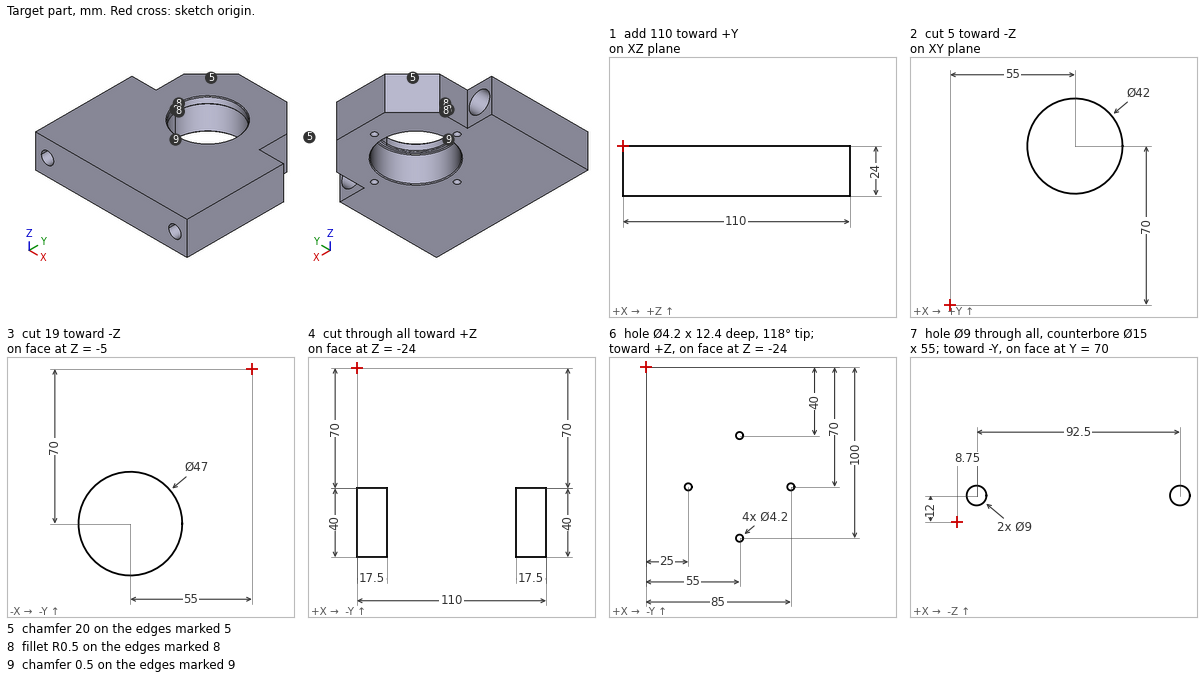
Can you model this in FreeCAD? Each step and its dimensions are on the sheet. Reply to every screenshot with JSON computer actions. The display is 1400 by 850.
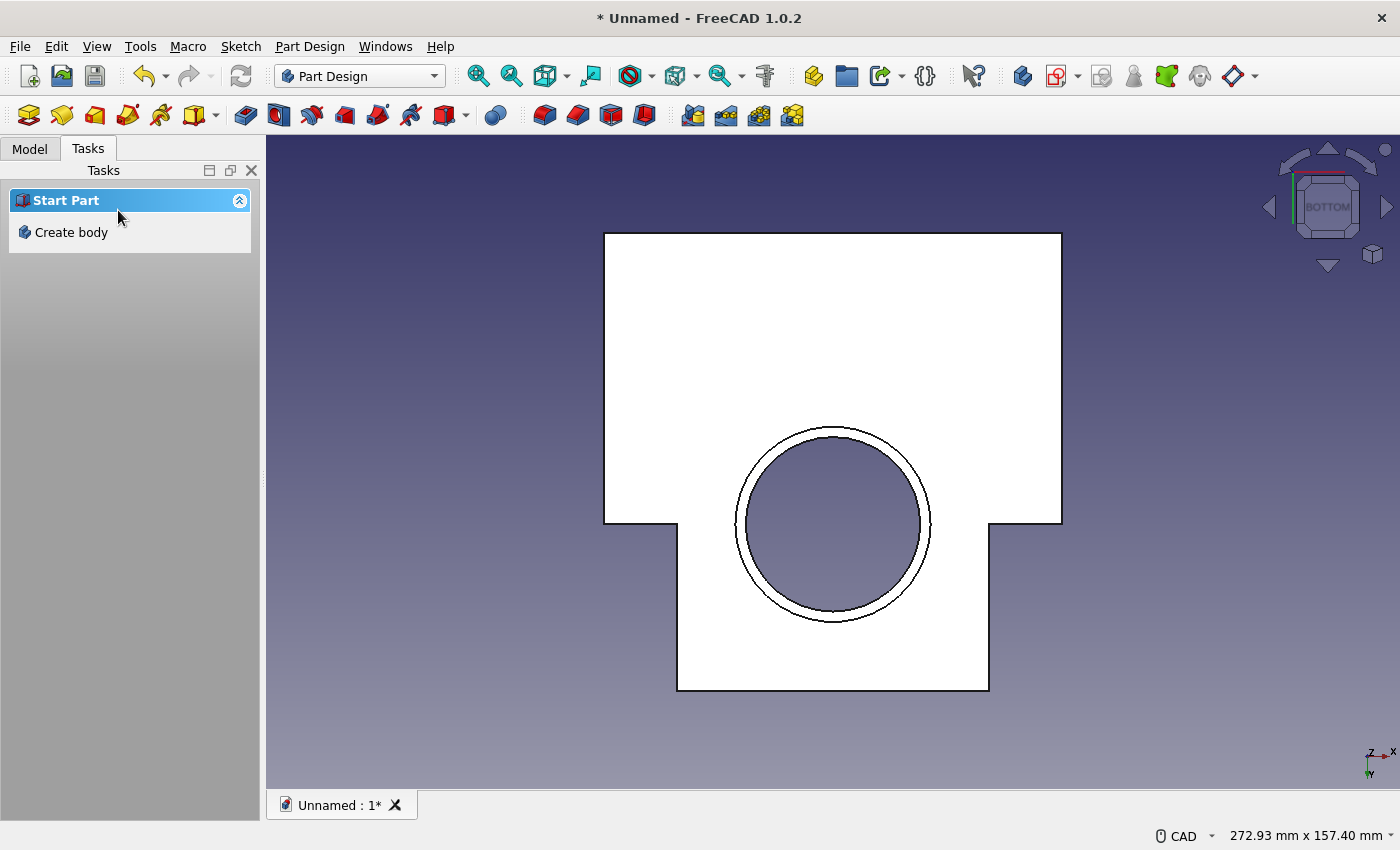
{"action": "key", "text": "0"}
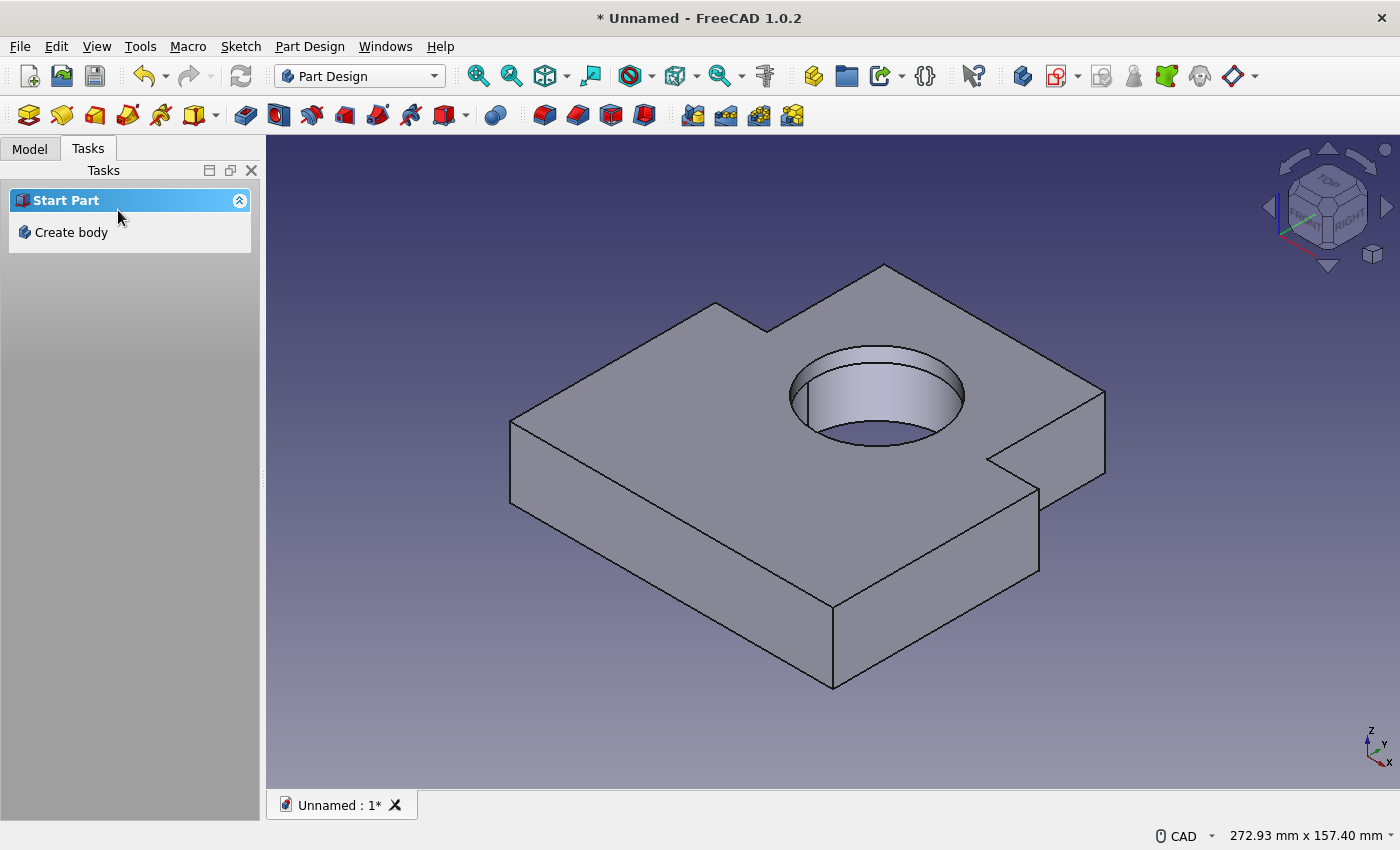
{"action": "key", "text": "2"}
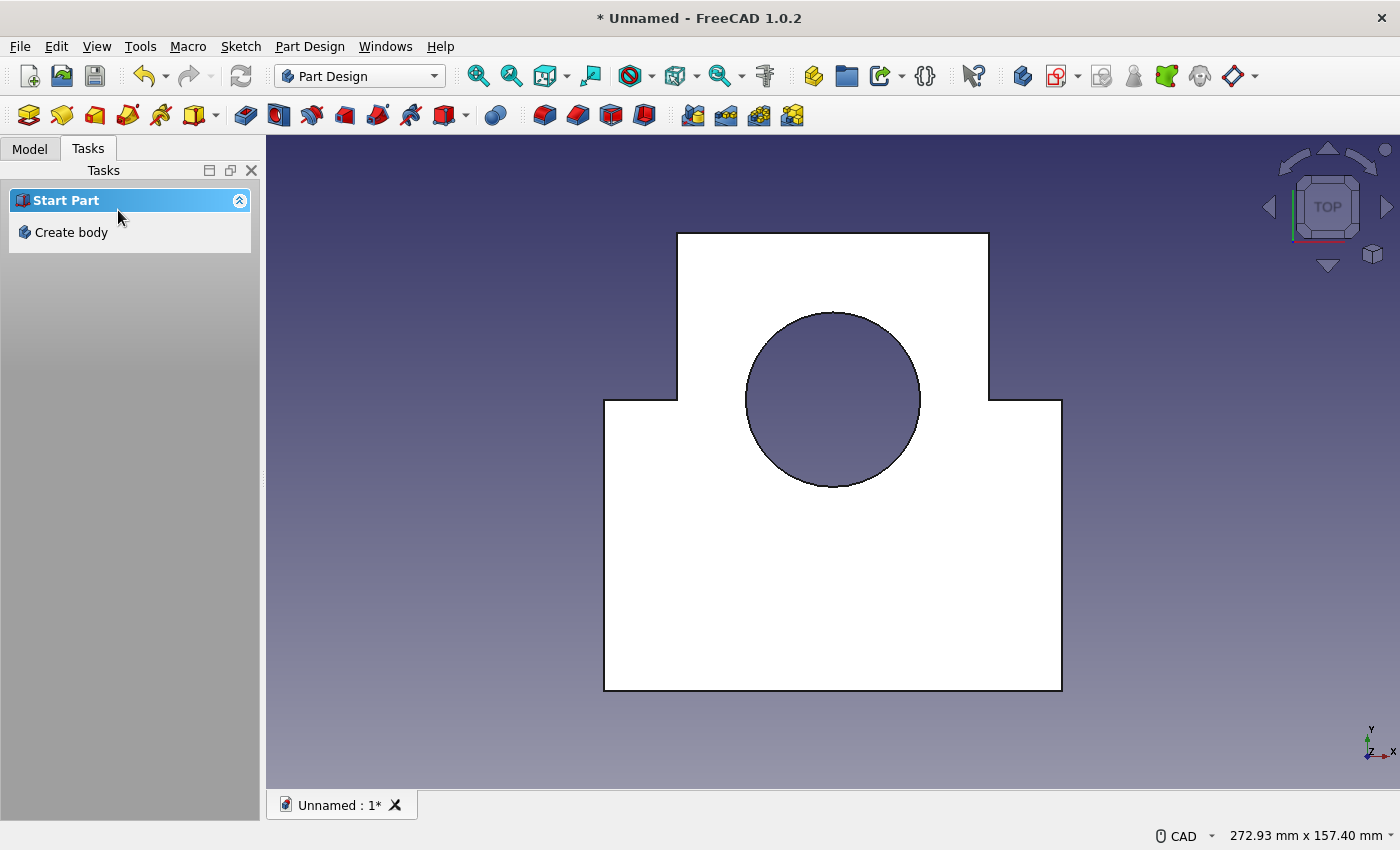
{"action": "key", "text": "1"}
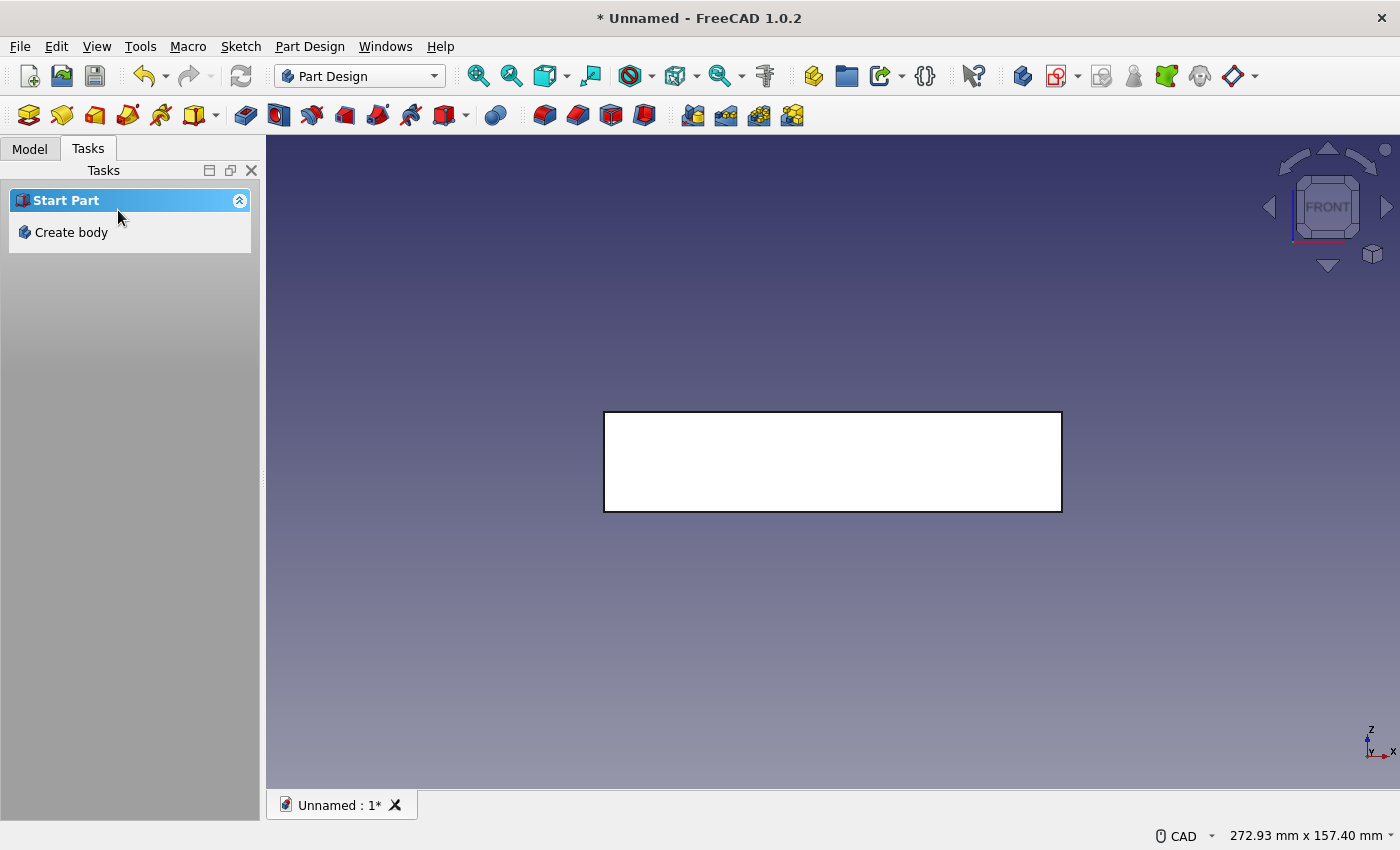
{"action": "left_click", "coordinate": [479, 76]}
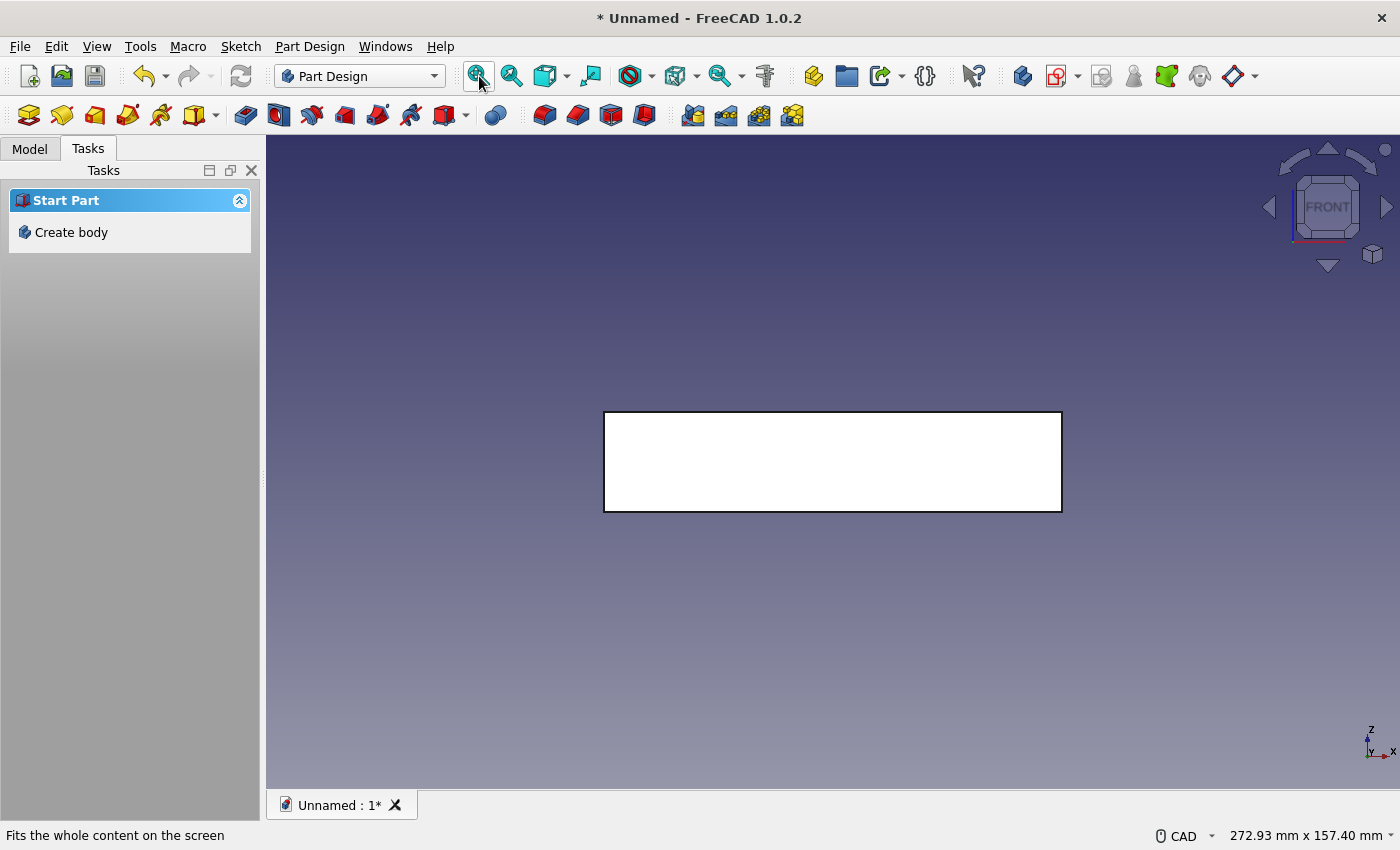
{"action": "key", "text": "3"}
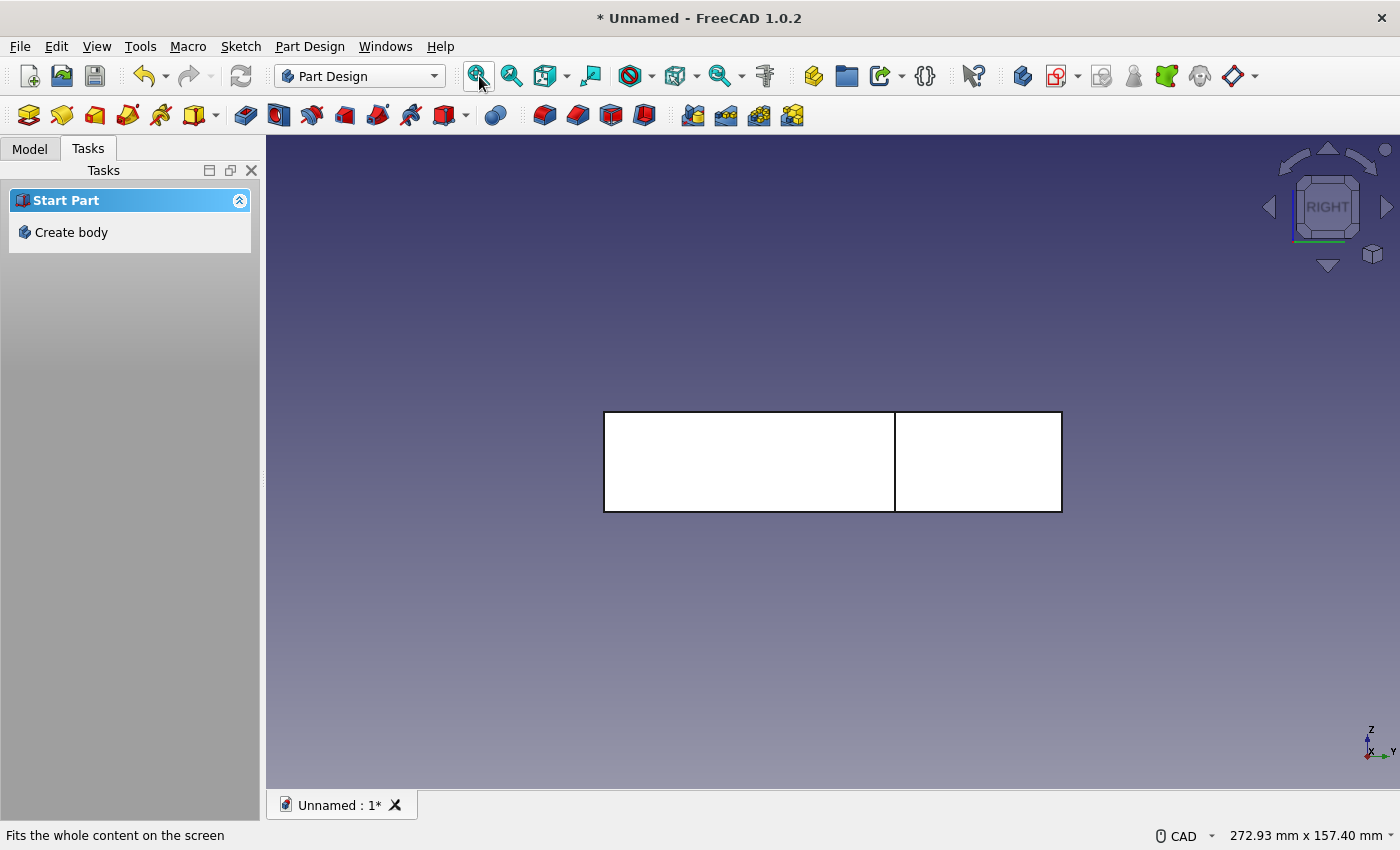
{"action": "left_click", "coordinate": [479, 76]}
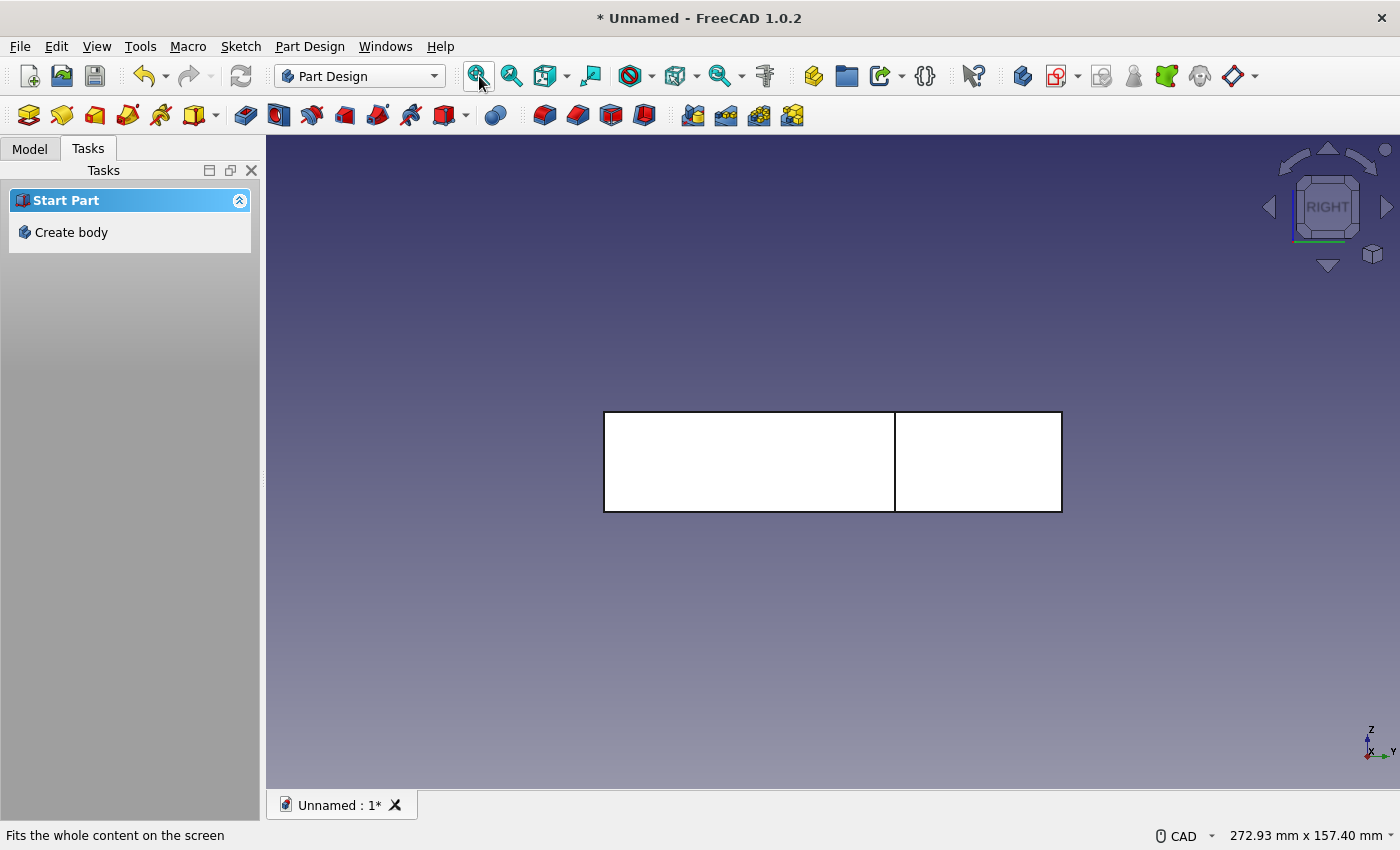
{"action": "left_click", "coordinate": [1062, 461]}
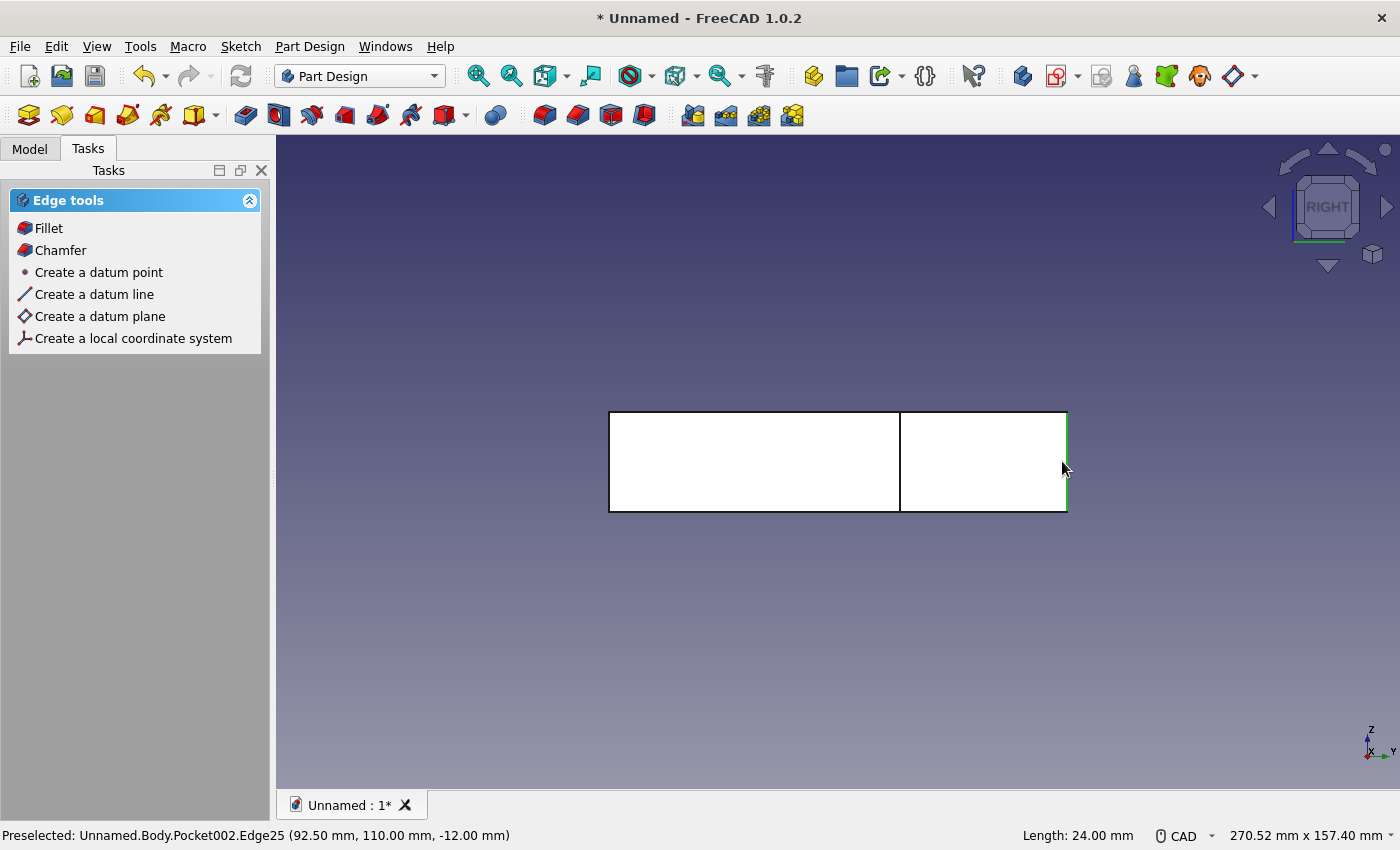
{"action": "key", "text": "5"}